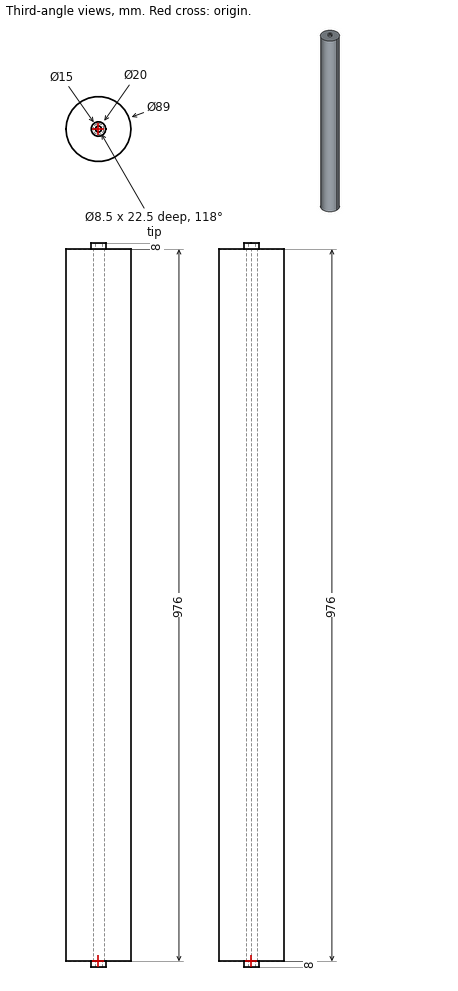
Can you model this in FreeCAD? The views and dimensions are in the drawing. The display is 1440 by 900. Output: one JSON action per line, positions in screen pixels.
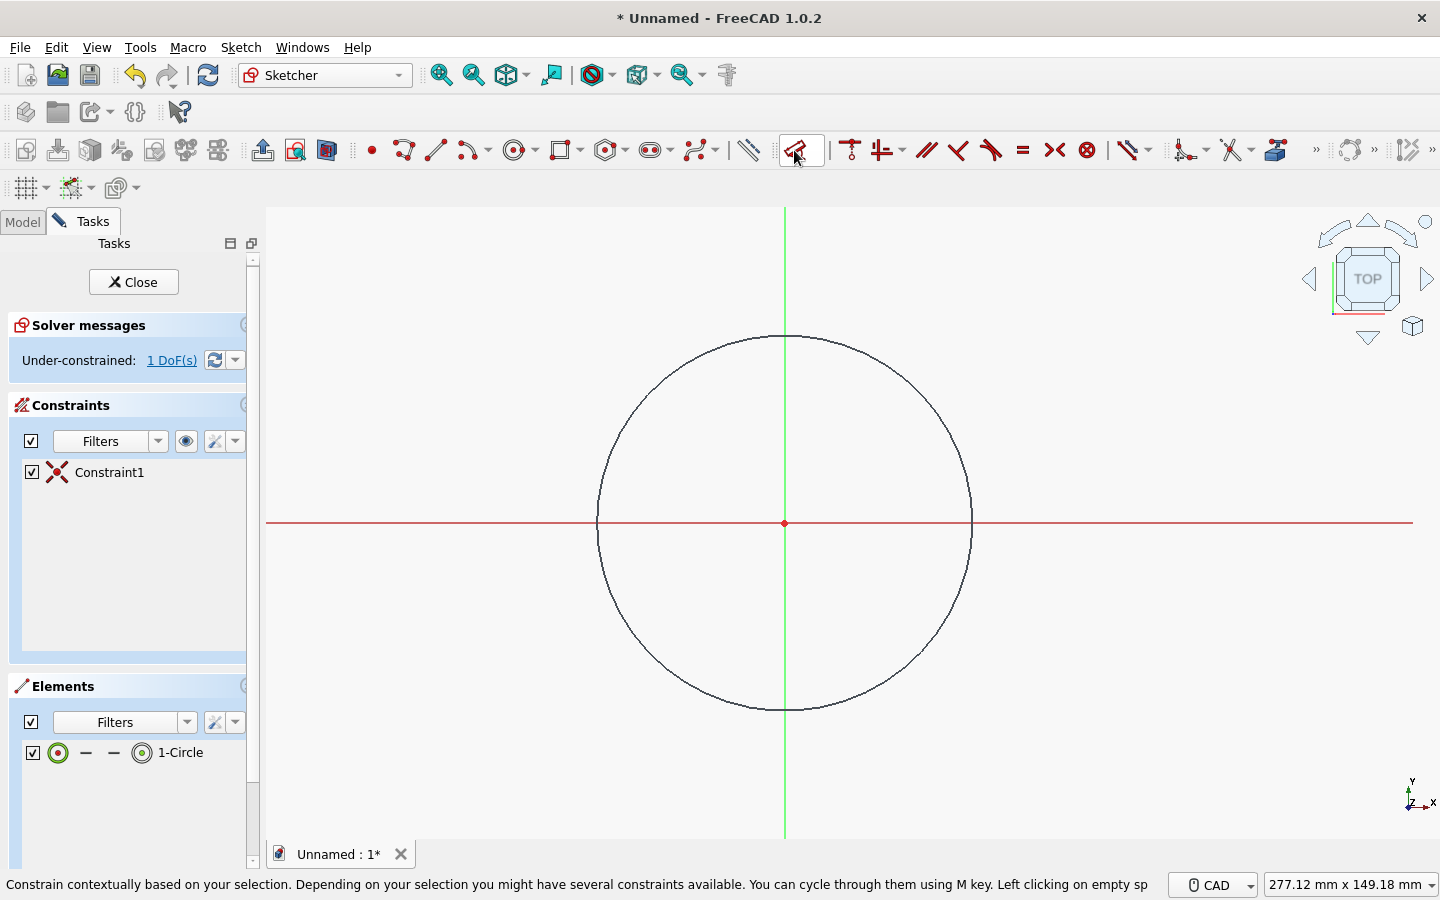
{"action": "left_click", "coordinate": [917, 390]}
{"action": "left_click", "coordinate": [940, 367]}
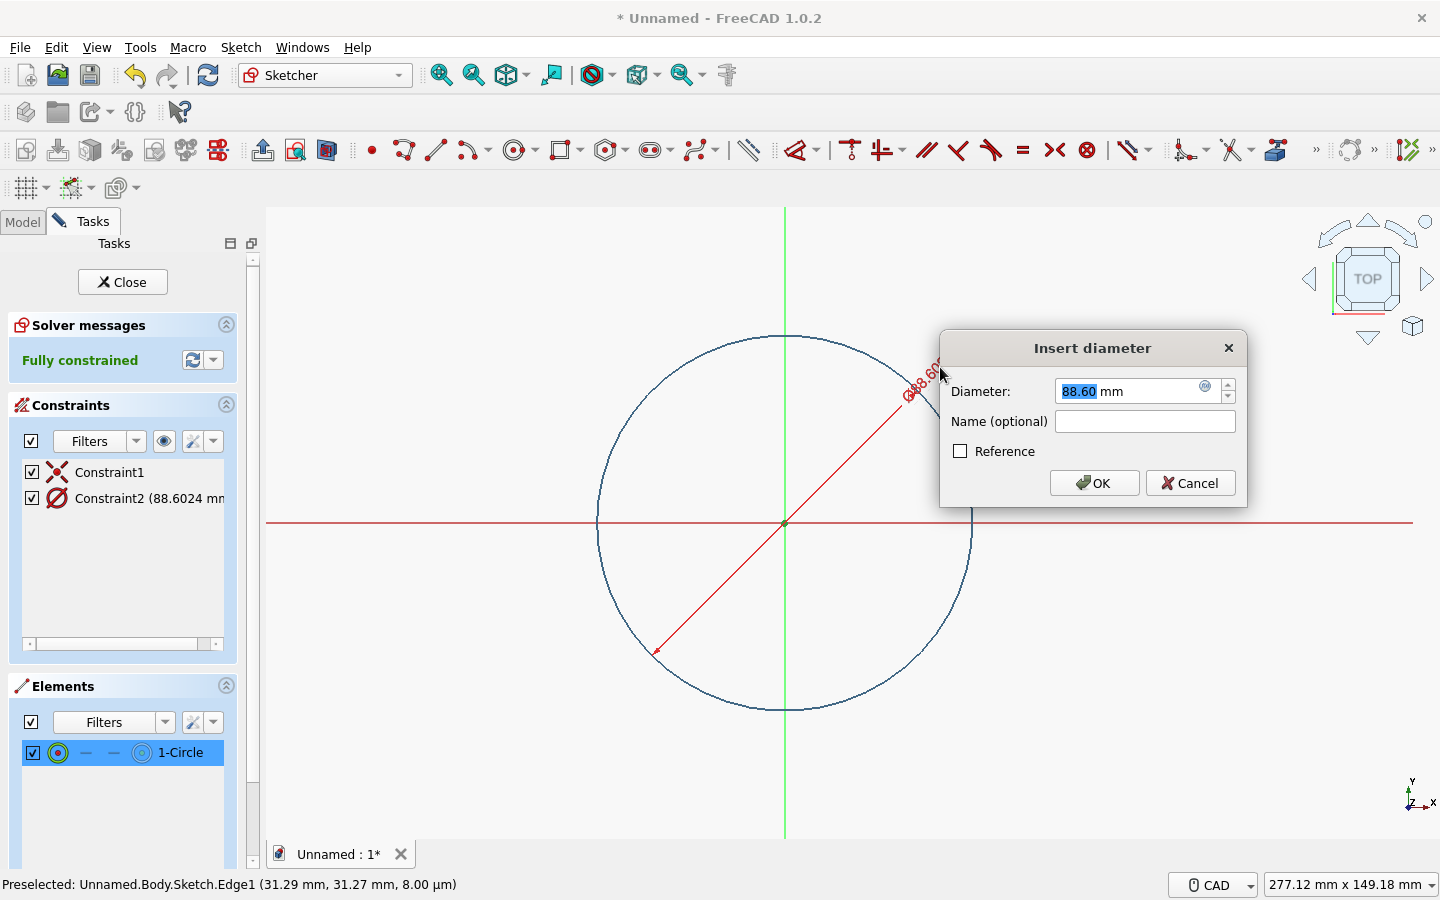
{"action": "type", "text": "89"}
{"action": "key", "text": "Return"}
{"action": "key", "text": "Escape"}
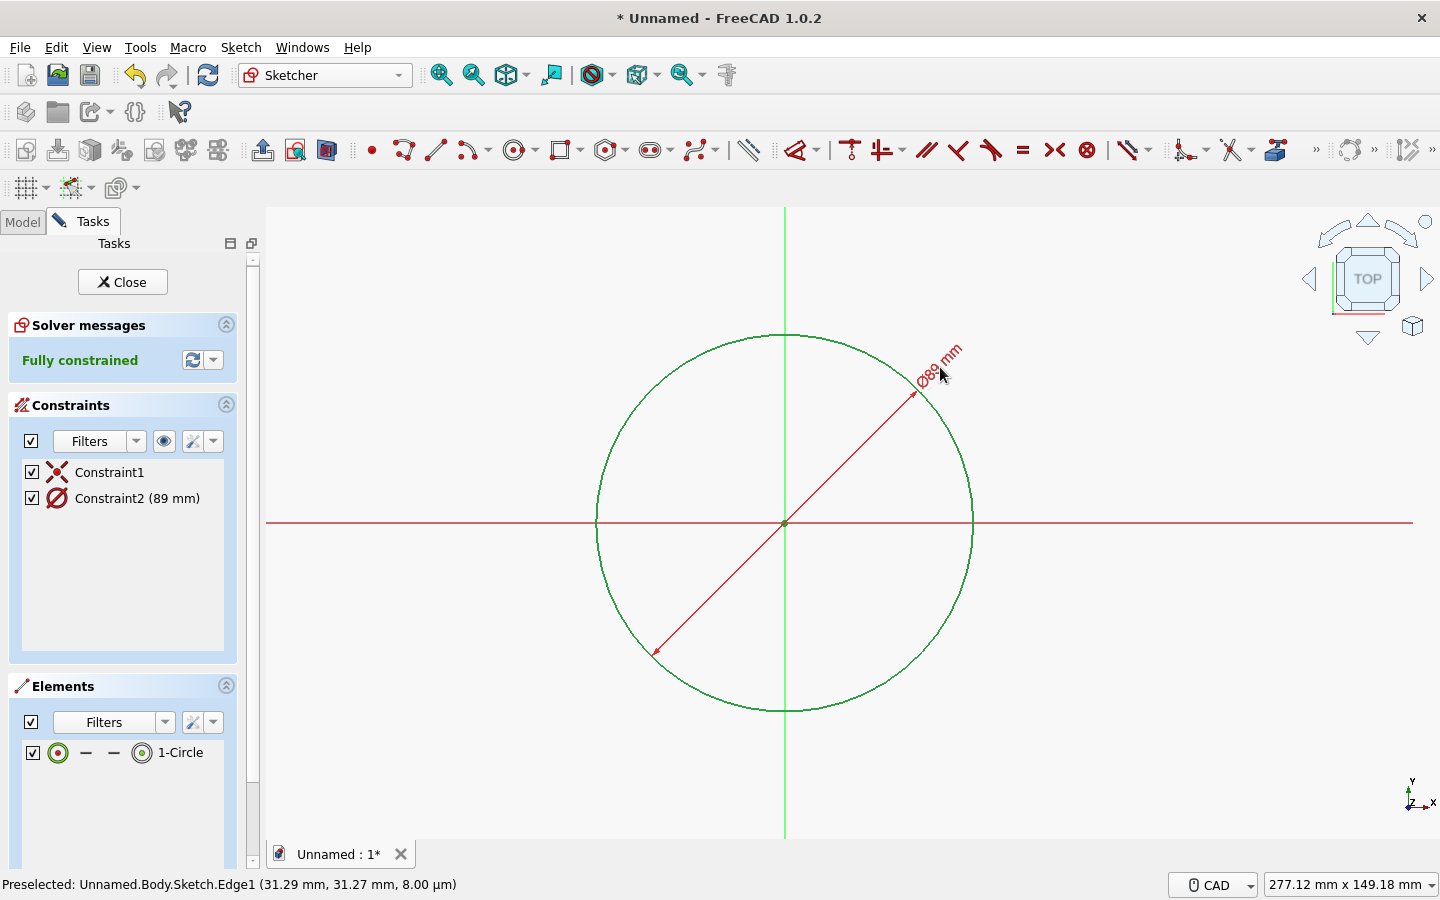
{"action": "left_click", "coordinate": [123, 282]}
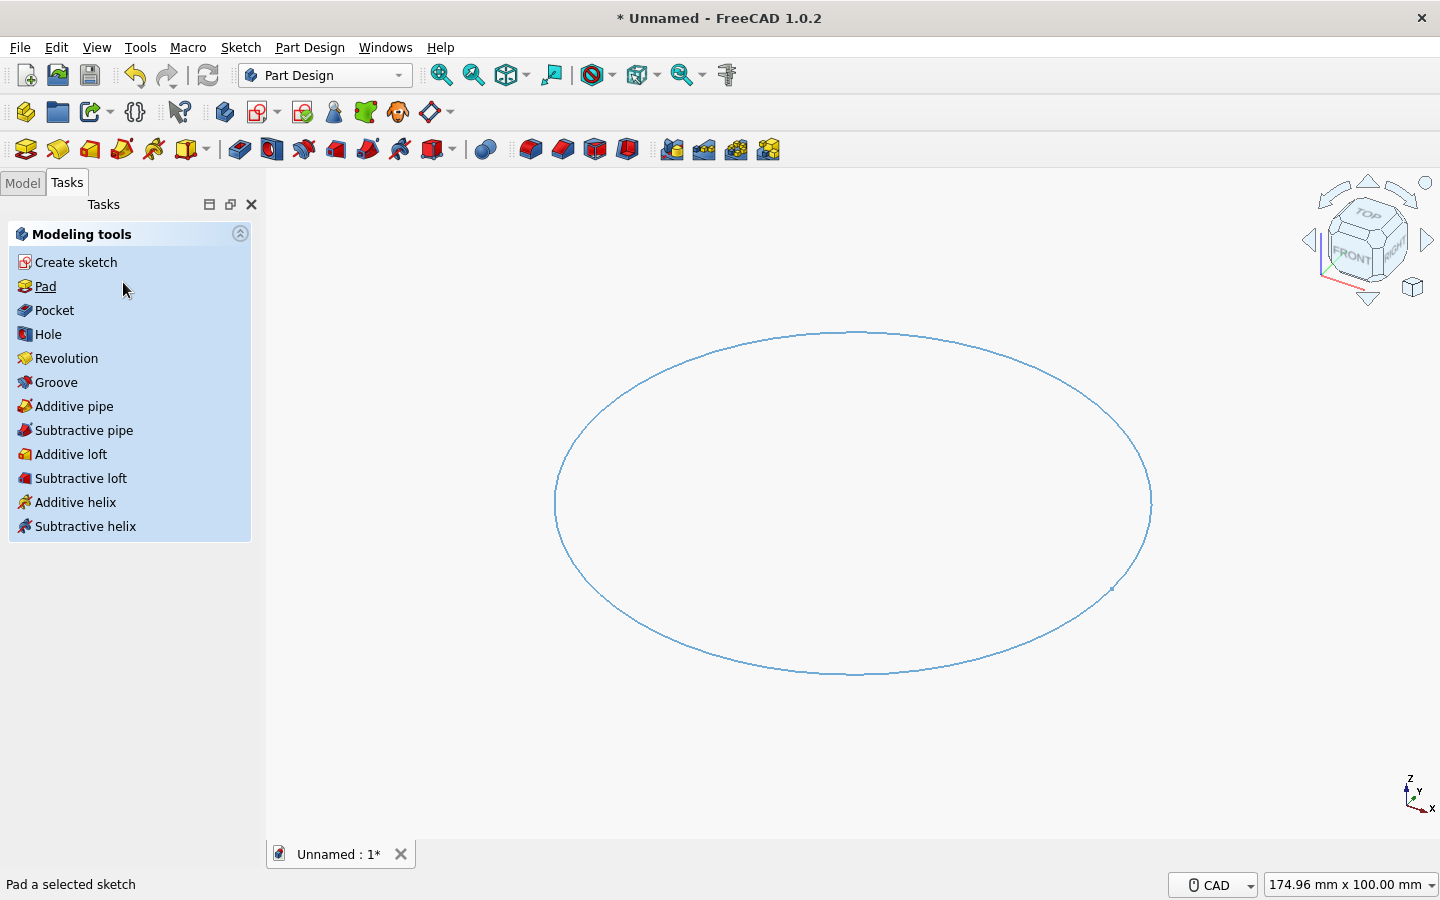
{"action": "left_click", "coordinate": [26, 150]}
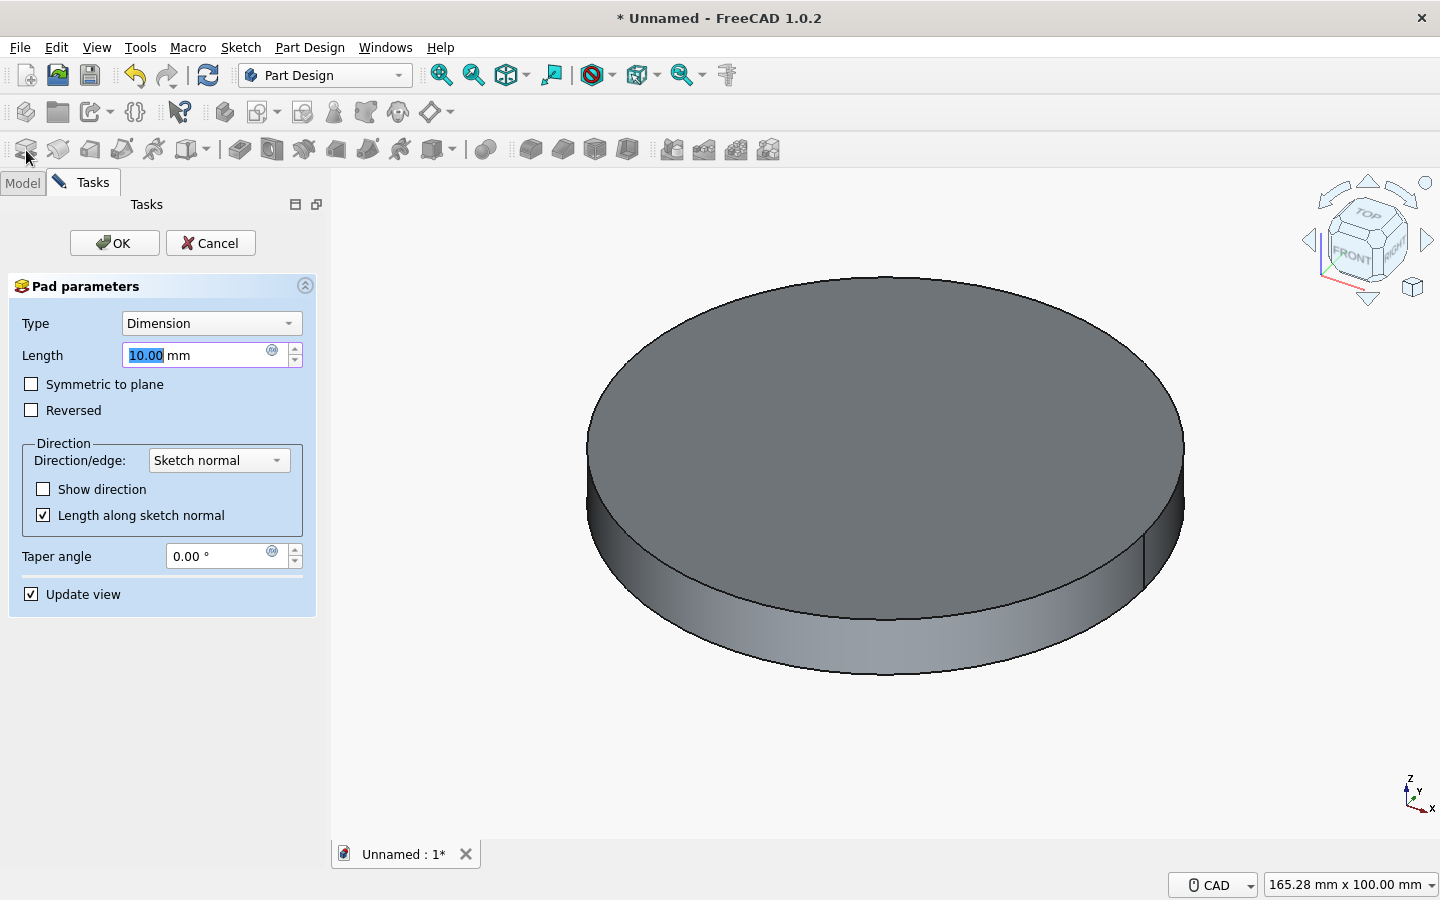
{"action": "type", "text": "976"}
{"action": "key", "text": "Tab"}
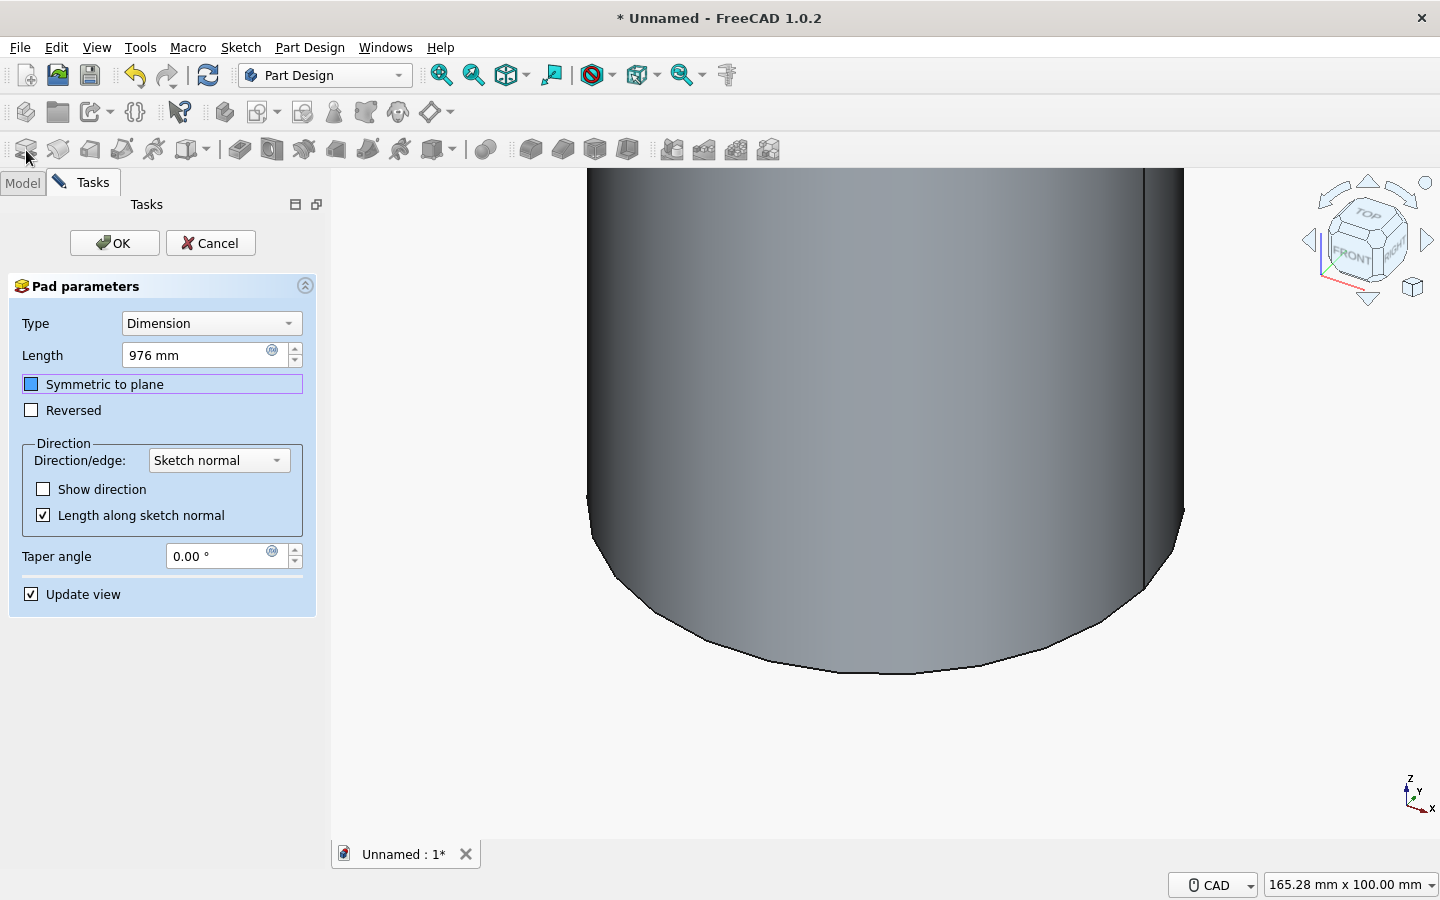
{"action": "left_click", "coordinate": [115, 243]}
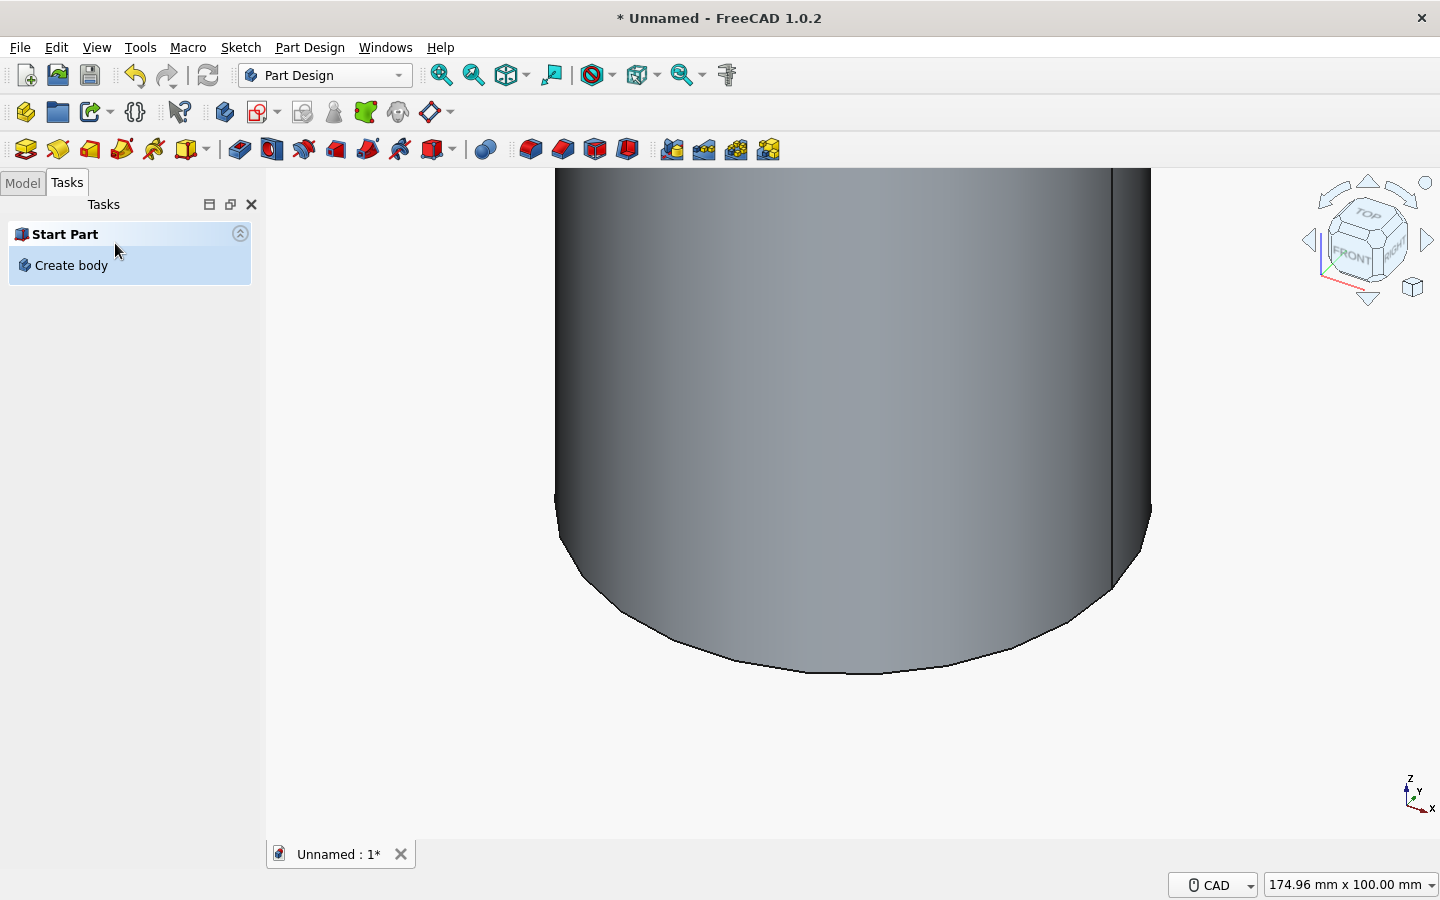
{"action": "left_click", "coordinate": [442, 76]}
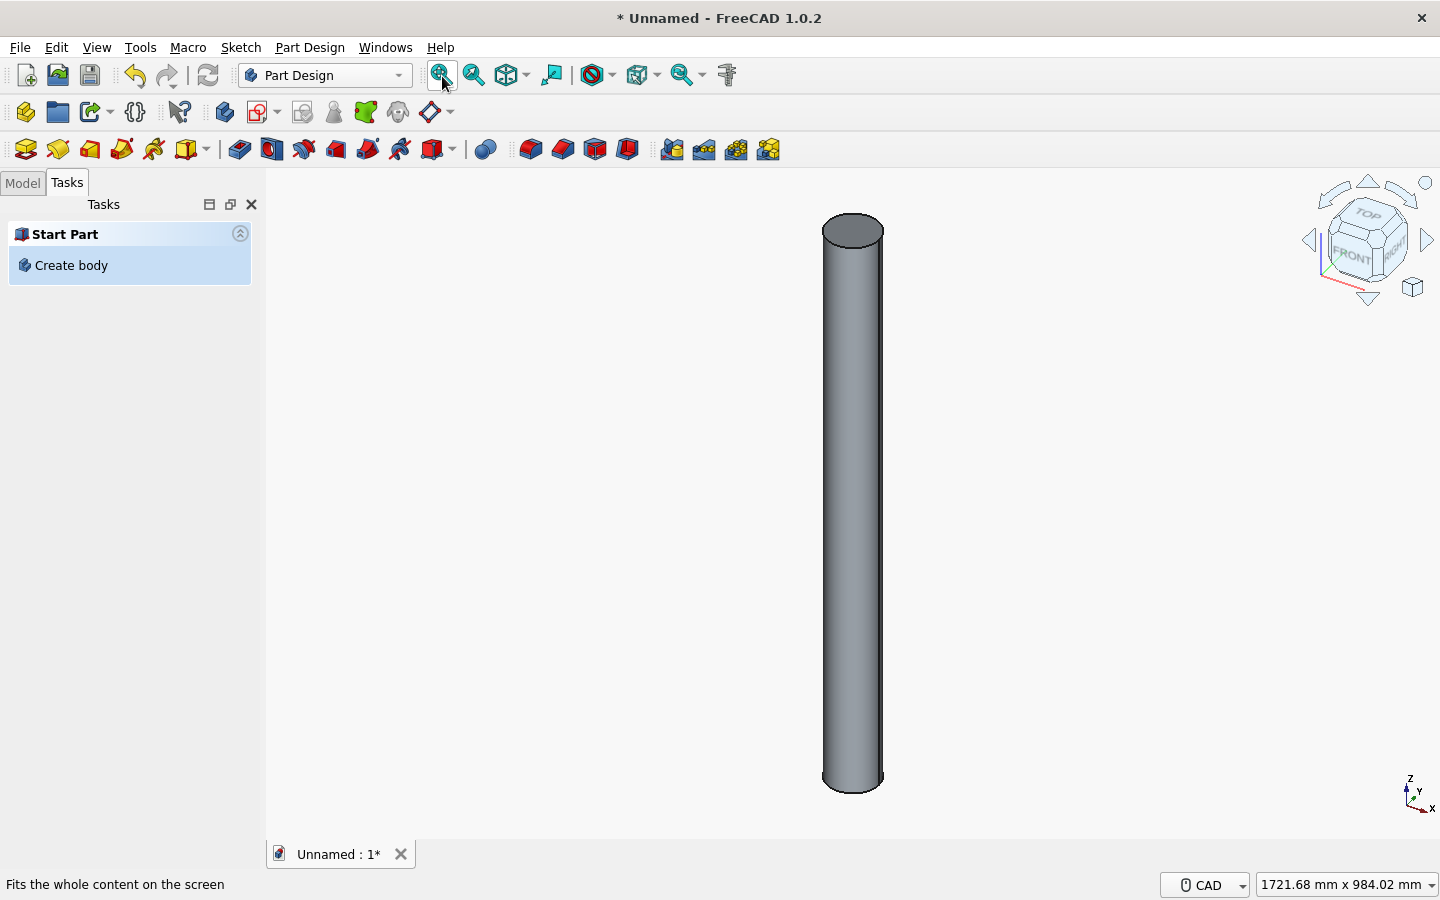
{"action": "left_click", "coordinate": [853, 230]}